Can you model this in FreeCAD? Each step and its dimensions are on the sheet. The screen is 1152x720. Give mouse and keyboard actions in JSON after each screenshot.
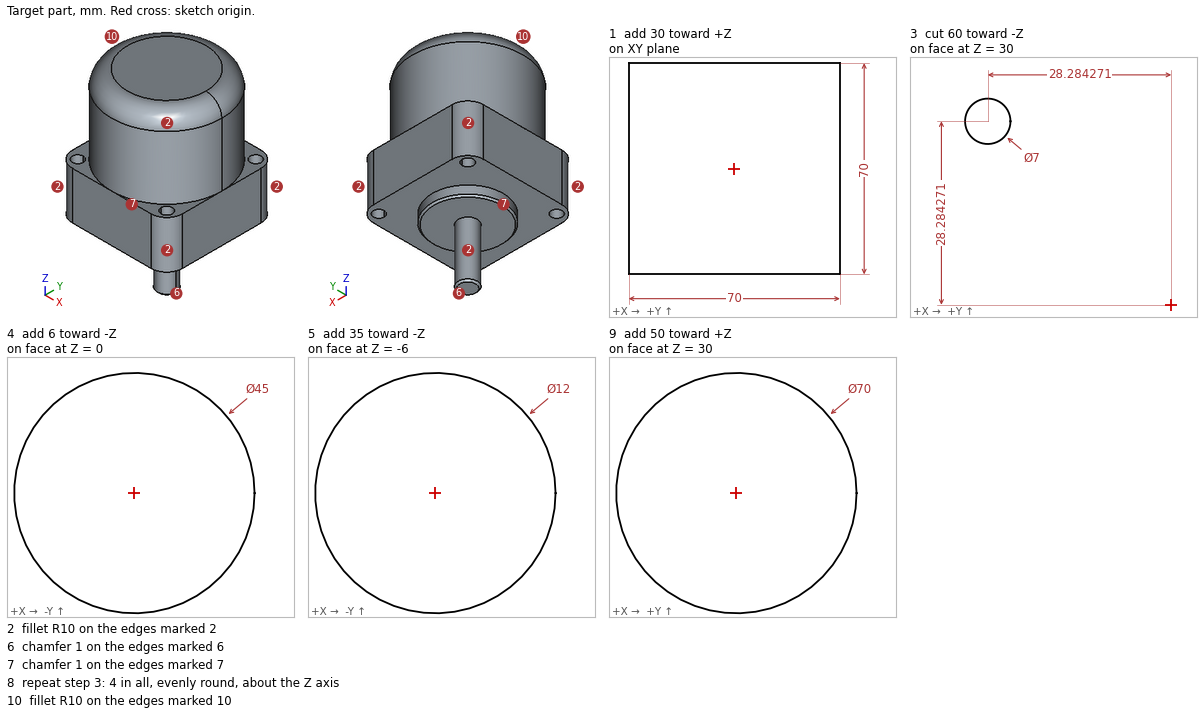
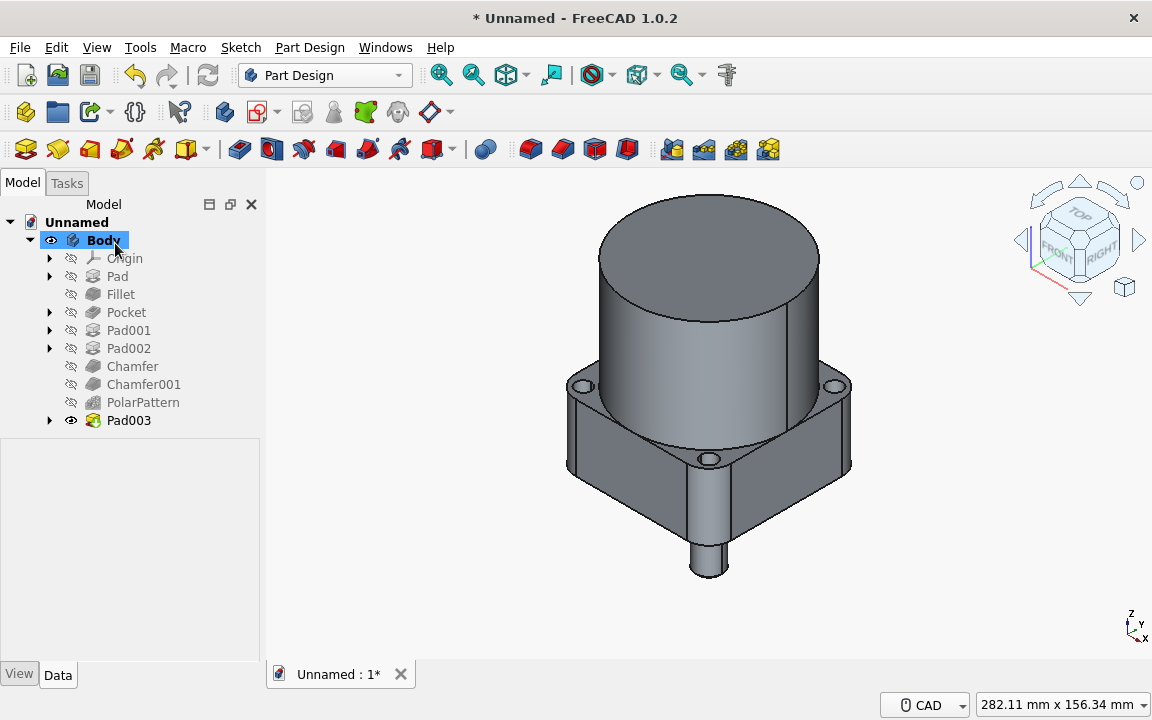
{"action": "left_click", "coordinate": [611, 286]}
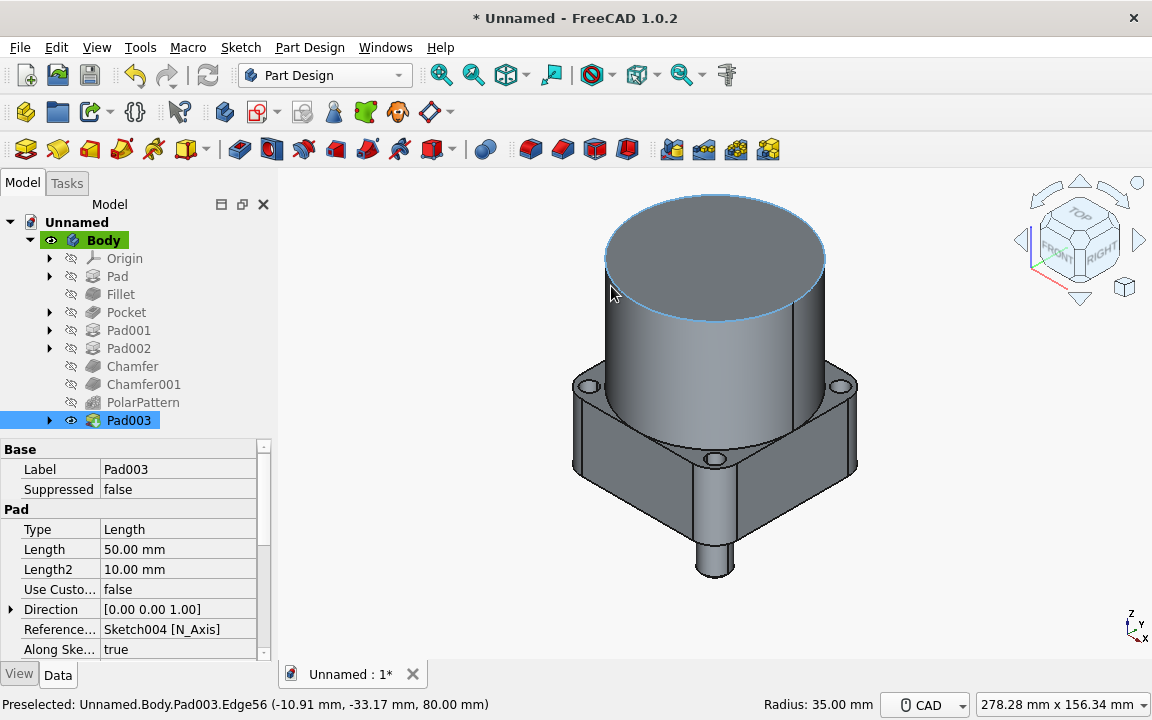
{"action": "left_click", "coordinate": [532, 150]}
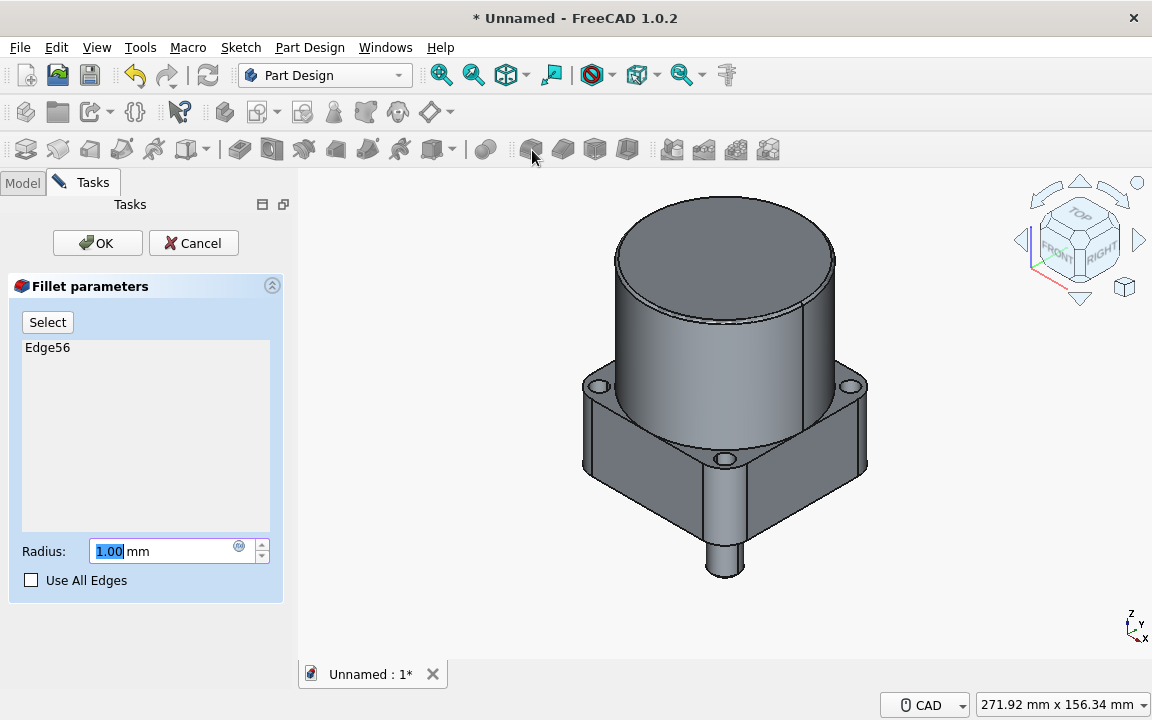
{"action": "type", "text": "10"}
{"action": "key", "text": "Tab"}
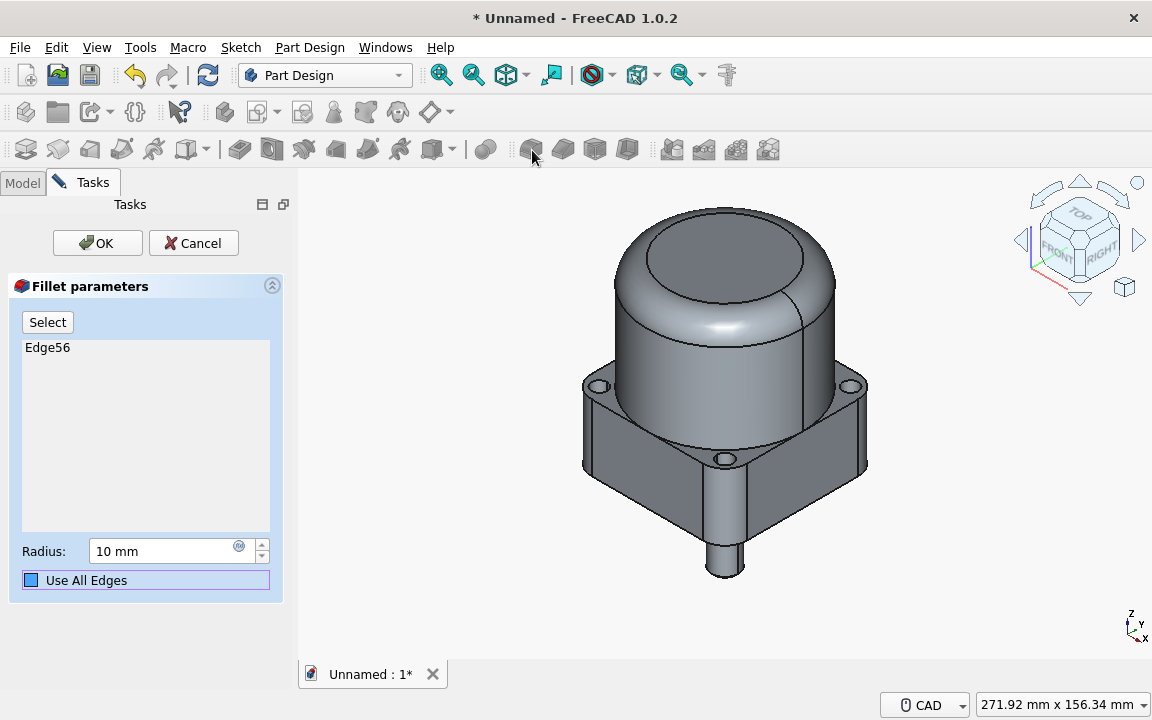
{"action": "left_click", "coordinate": [98, 243]}